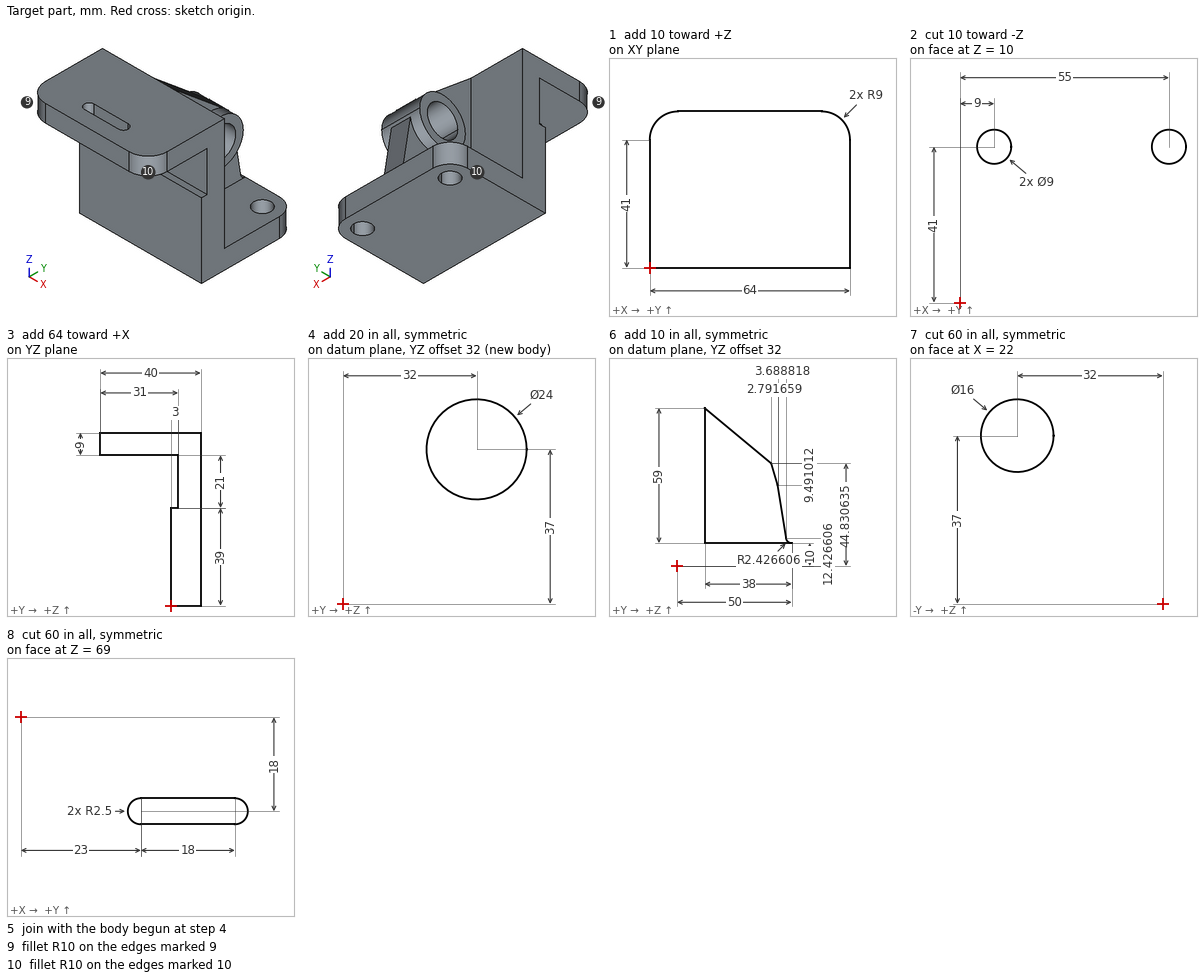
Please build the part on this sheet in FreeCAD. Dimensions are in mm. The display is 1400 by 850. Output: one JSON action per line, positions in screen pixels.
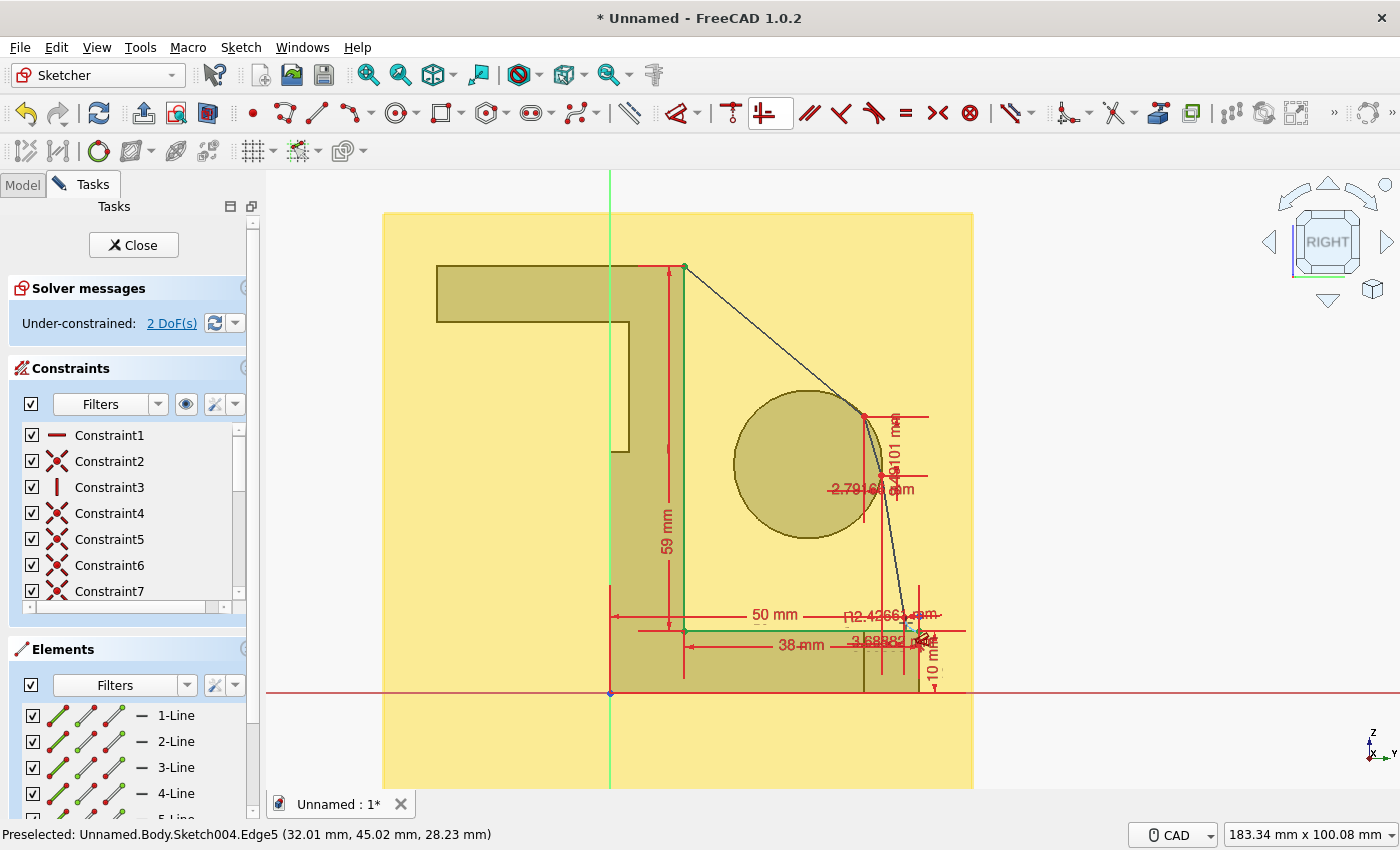
{"action": "left_click", "coordinate": [864, 417]}
{"action": "left_click", "coordinate": [576, 555]}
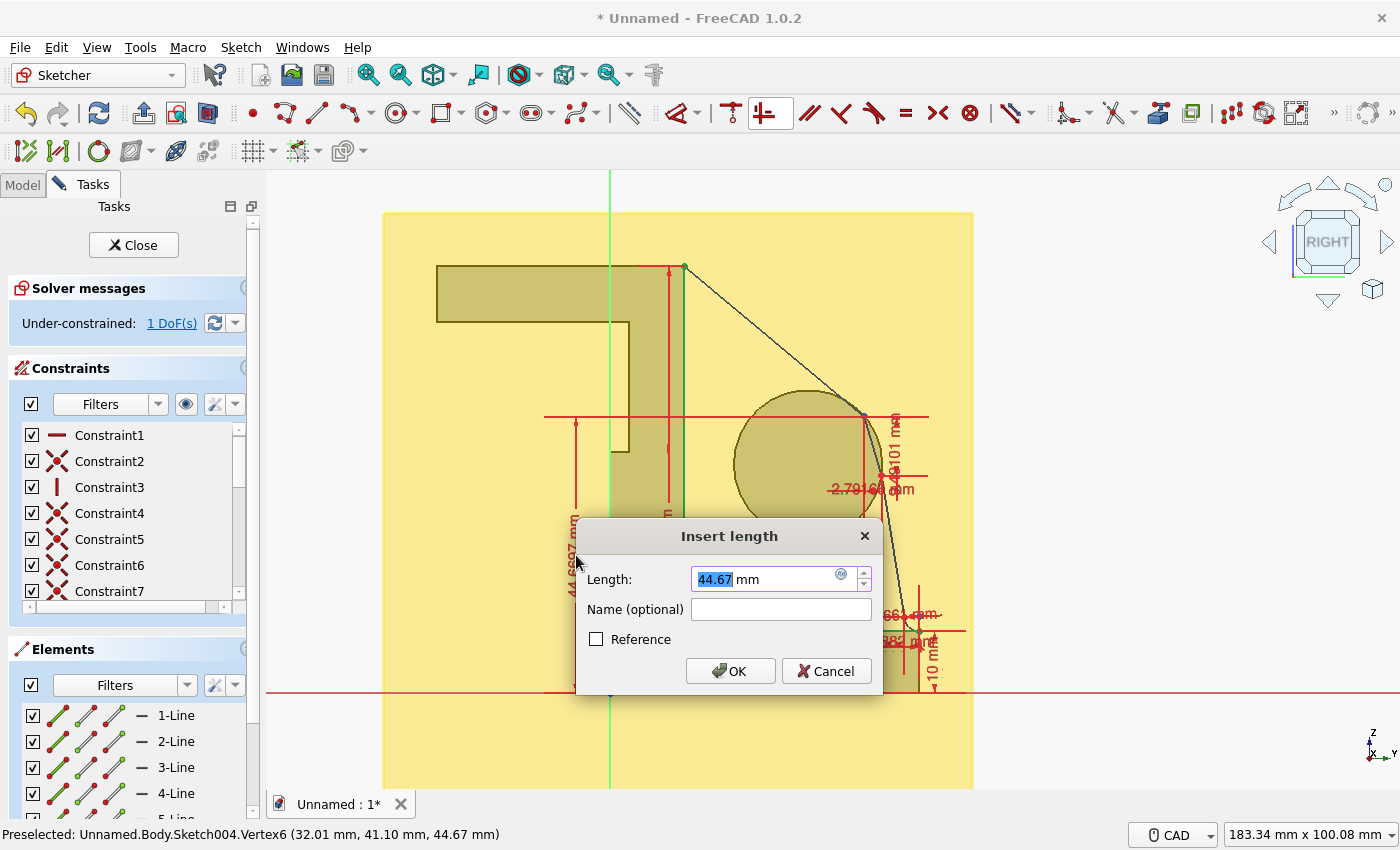
{"action": "type", "text": "44.830635"}
{"action": "key", "text": "Return"}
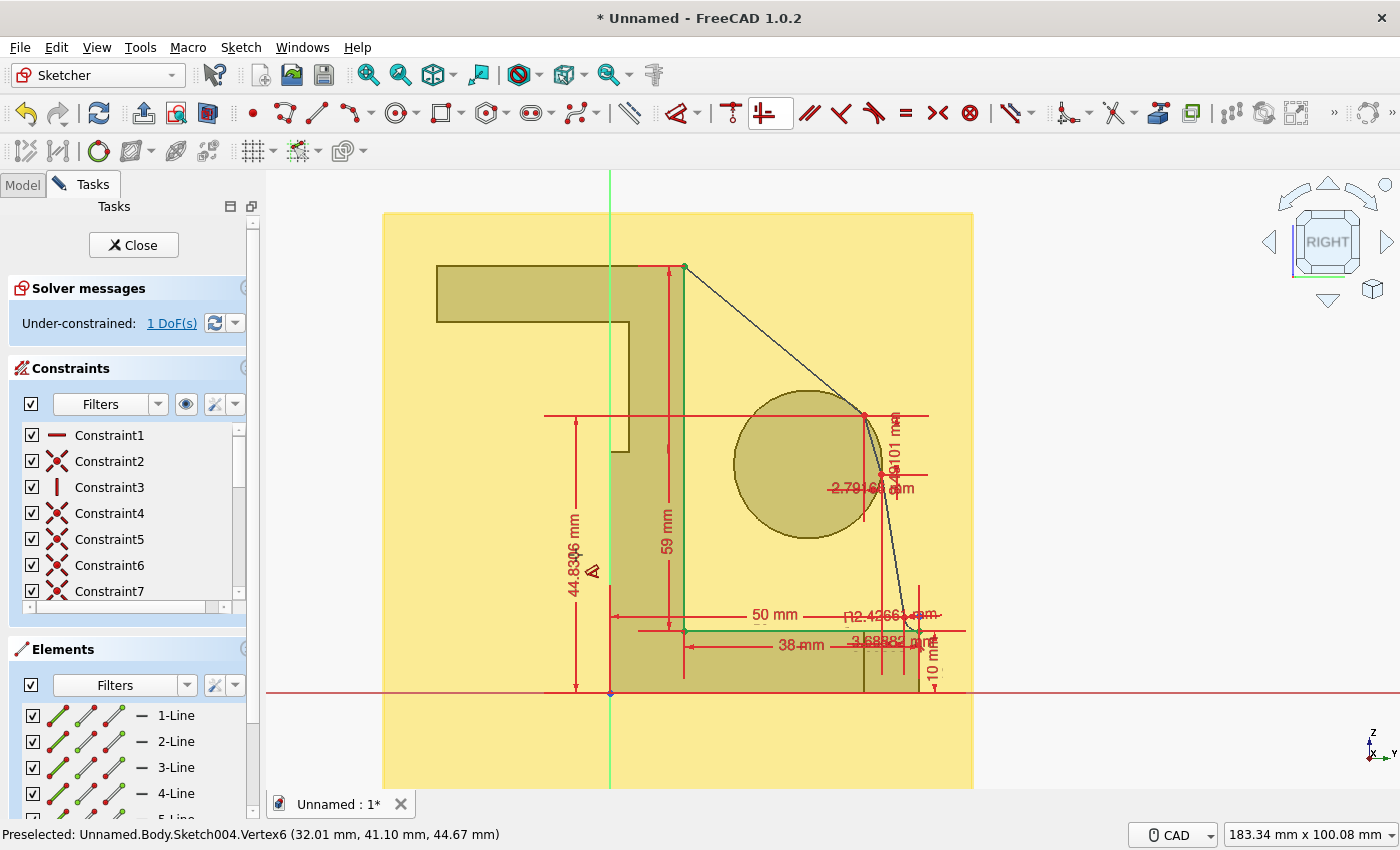
{"action": "left_click", "coordinate": [904, 617]}
{"action": "left_click", "coordinate": [576, 655]}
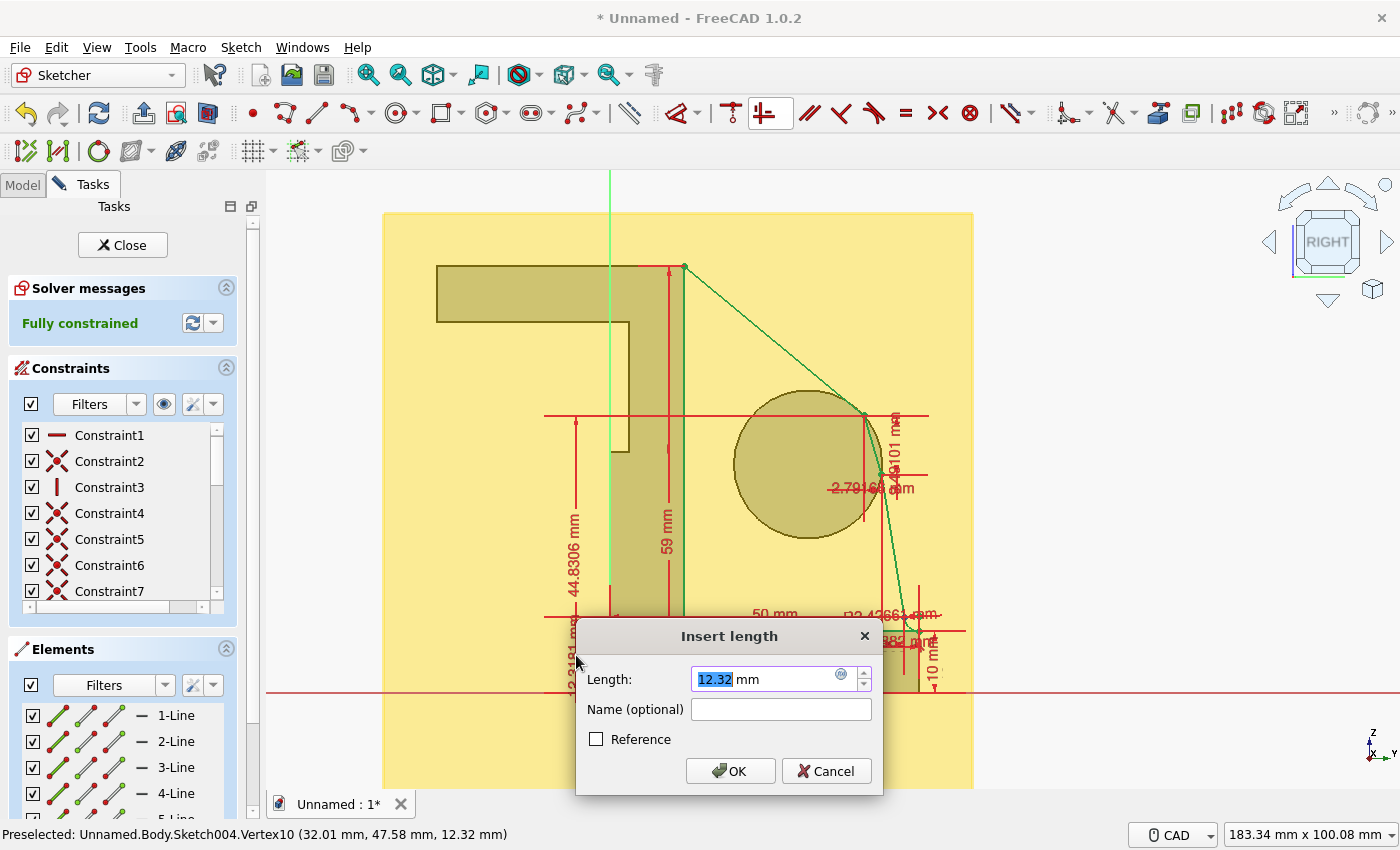
{"action": "type", "text": "12.426606"}
{"action": "key", "text": "Return"}
{"action": "key", "text": "Escape"}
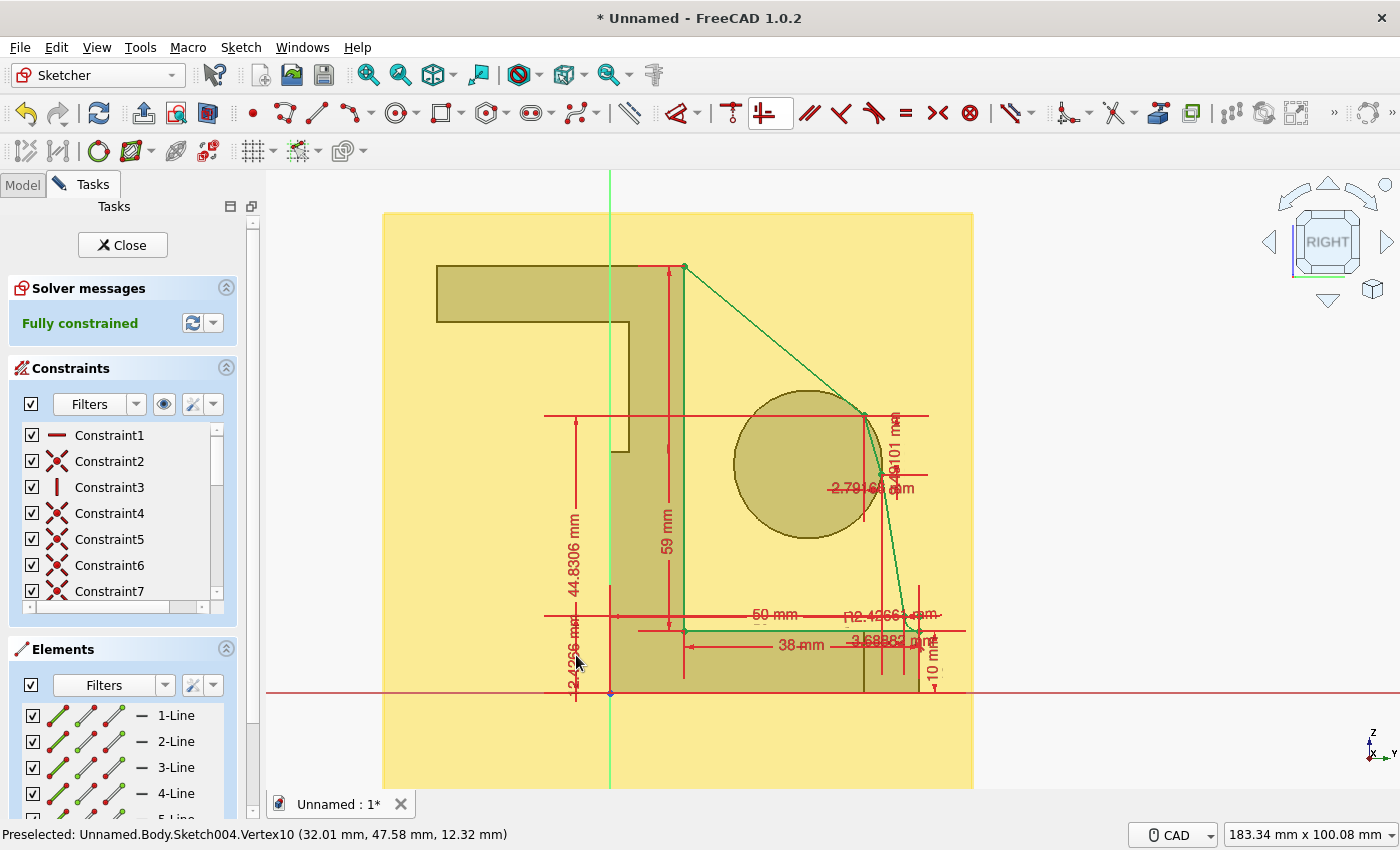
{"action": "left_click", "coordinate": [123, 245]}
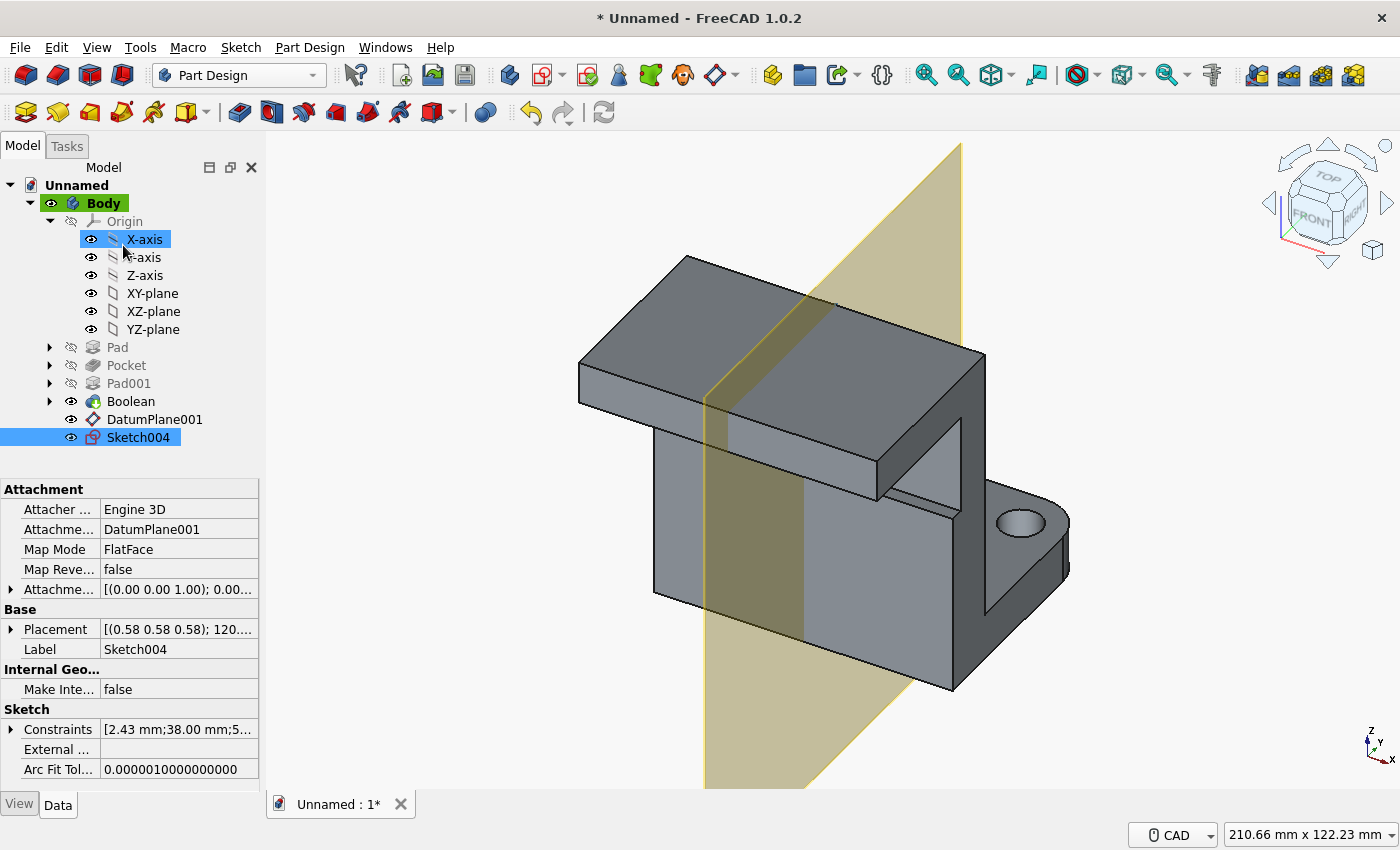
{"action": "left_click", "coordinate": [26, 112]}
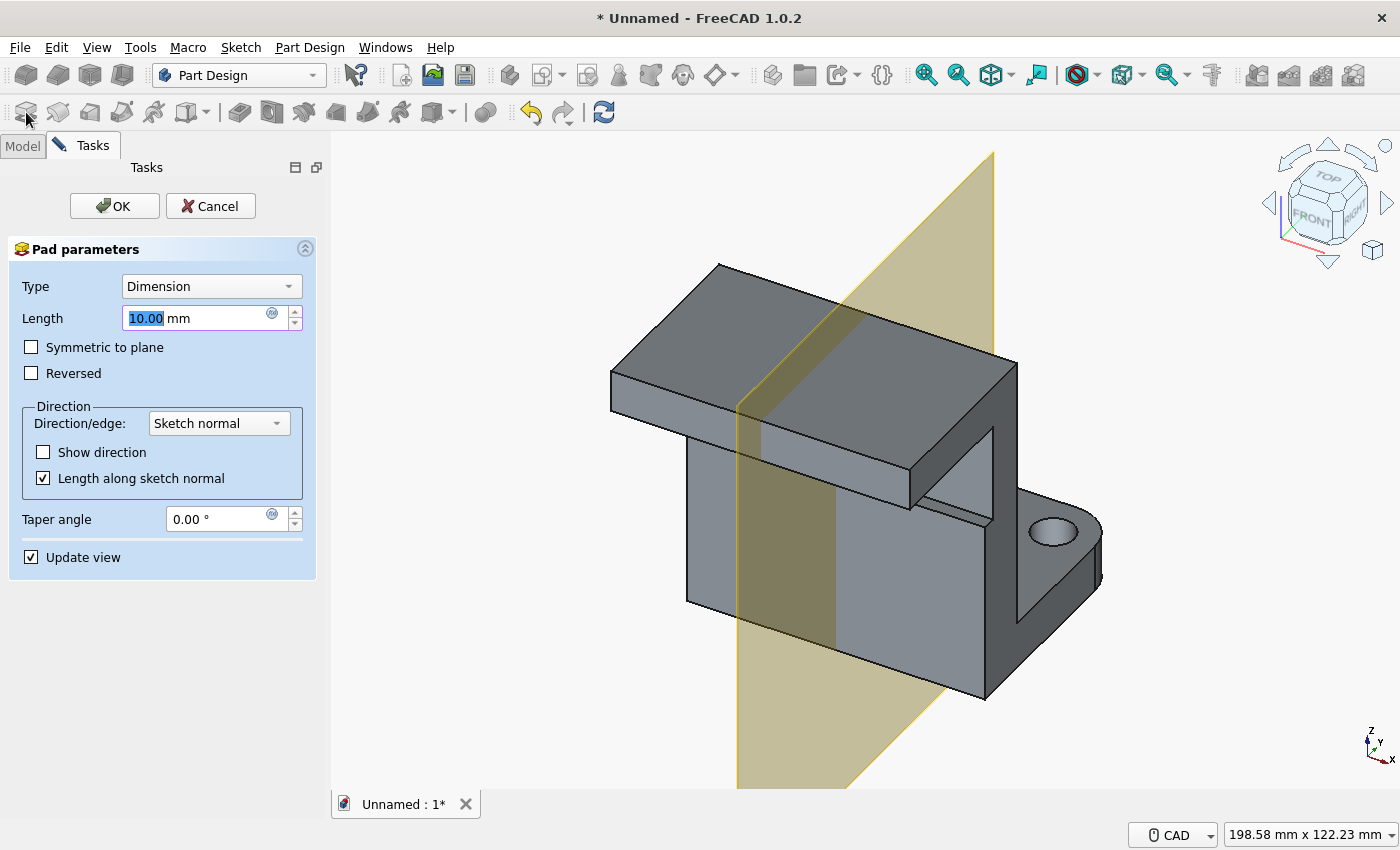
{"action": "type", "text": "10"}
{"action": "key", "text": "Tab"}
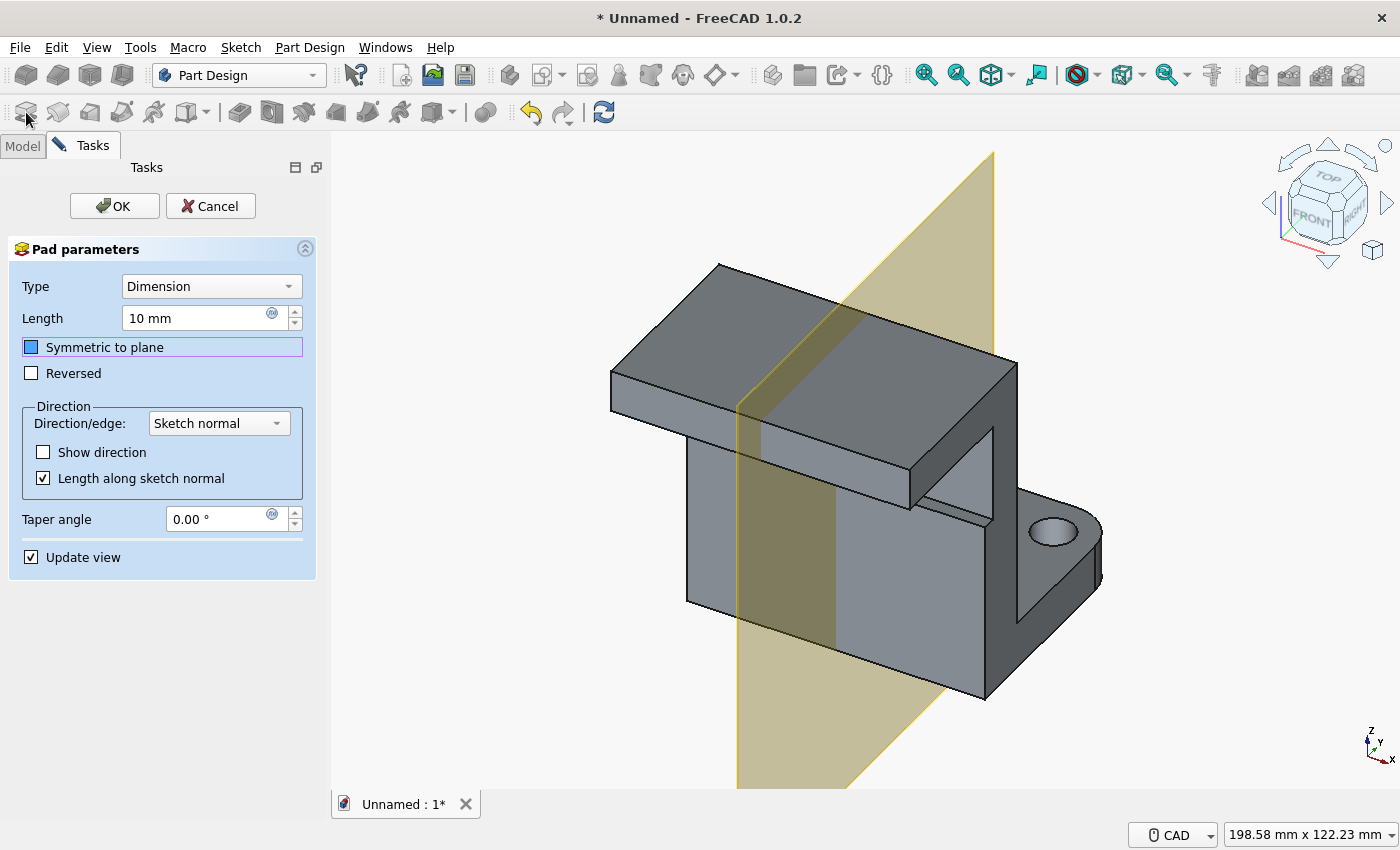
{"action": "left_click", "coordinate": [30, 347]}